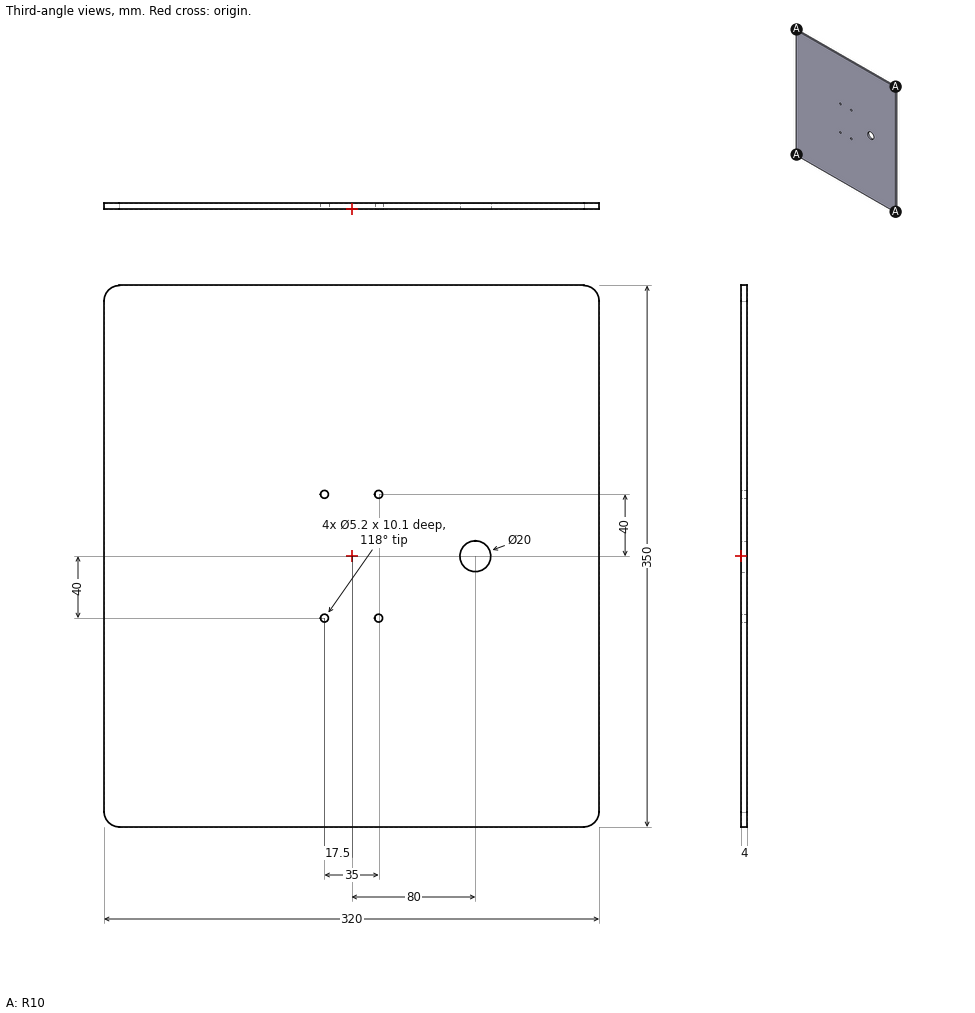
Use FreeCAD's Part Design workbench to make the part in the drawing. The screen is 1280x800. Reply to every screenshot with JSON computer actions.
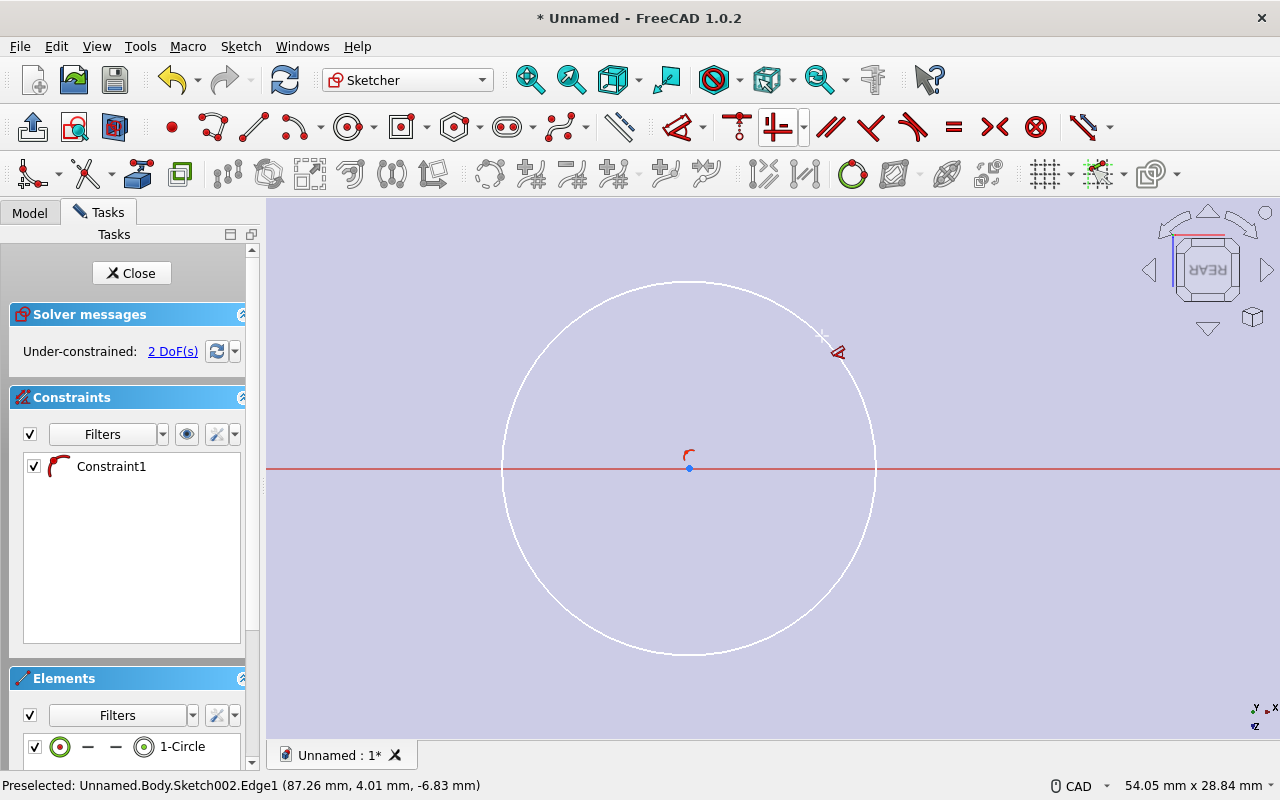
{"action": "left_click", "coordinate": [821, 336]}
{"action": "left_click", "coordinate": [844, 313]}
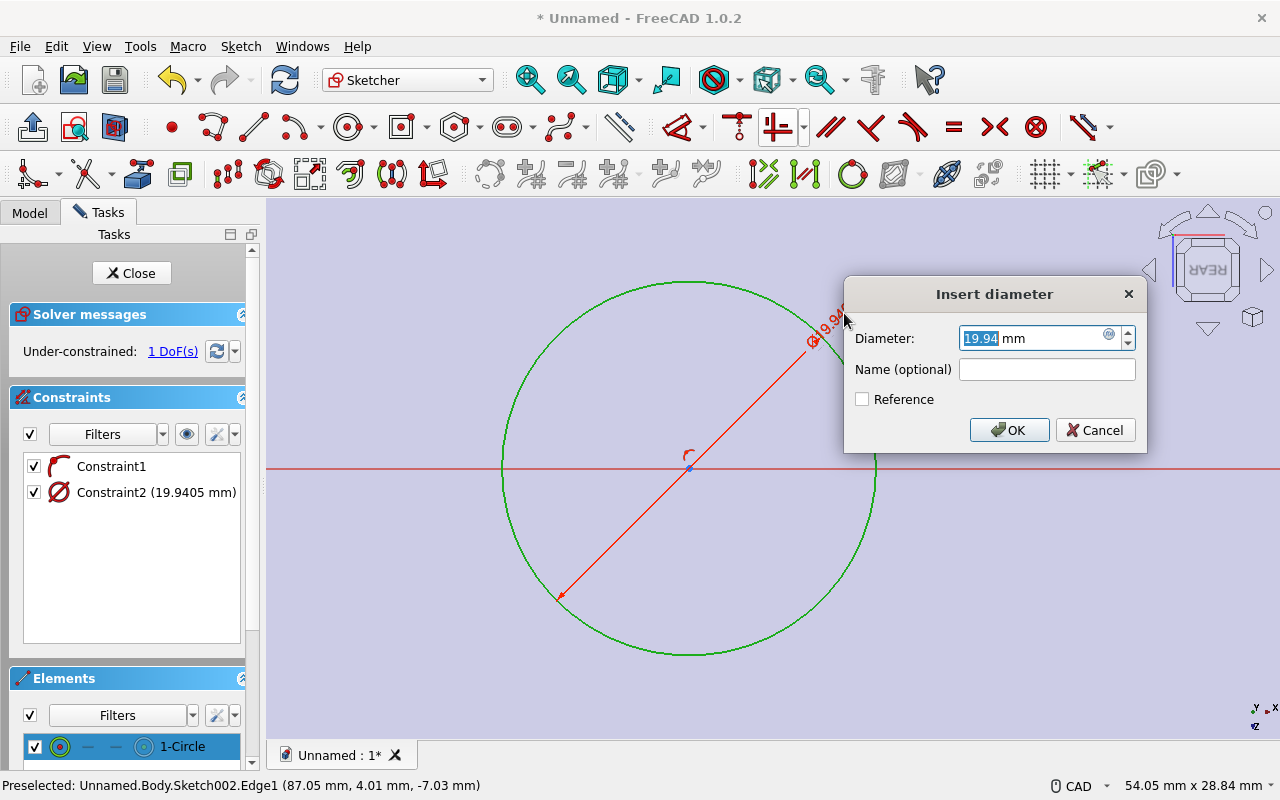
{"action": "type", "text": "20"}
{"action": "key", "text": "Return"}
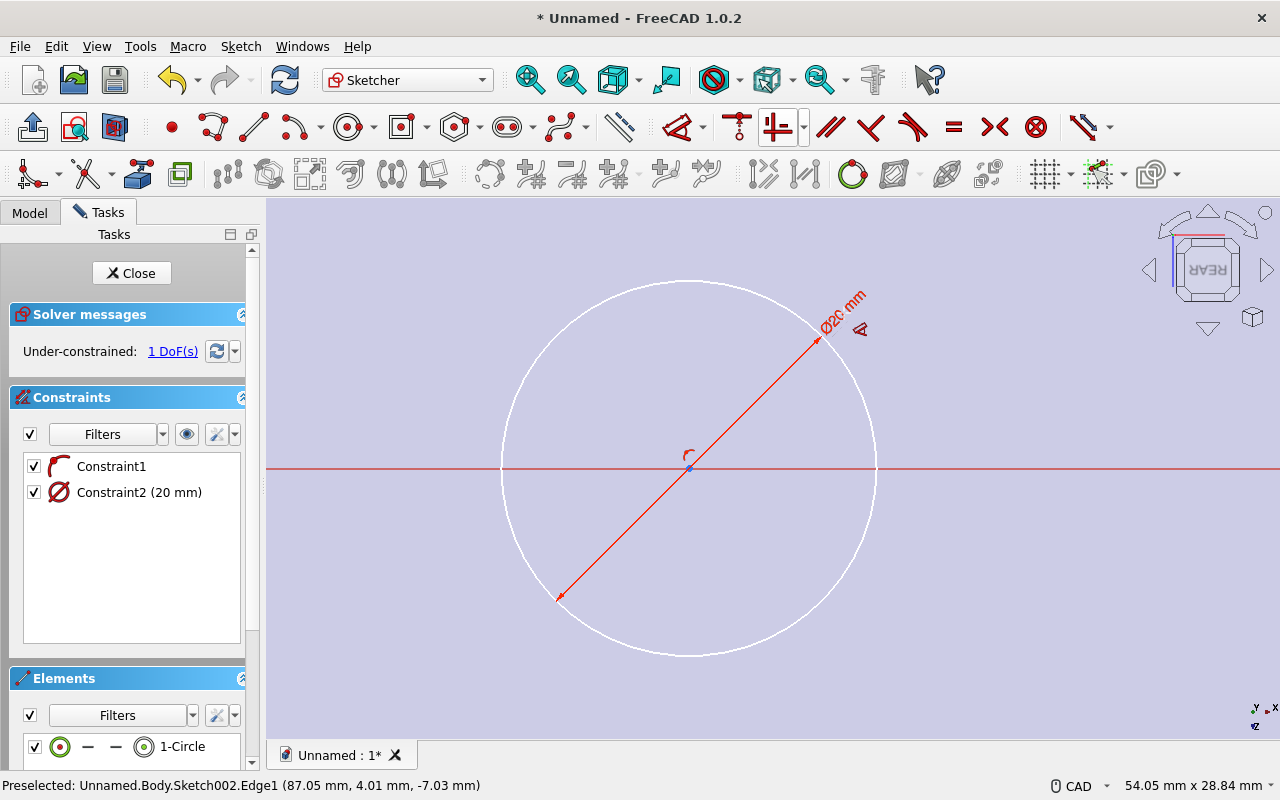
{"action": "left_click", "coordinate": [689, 468]}
{"action": "left_click", "coordinate": [401, 502]}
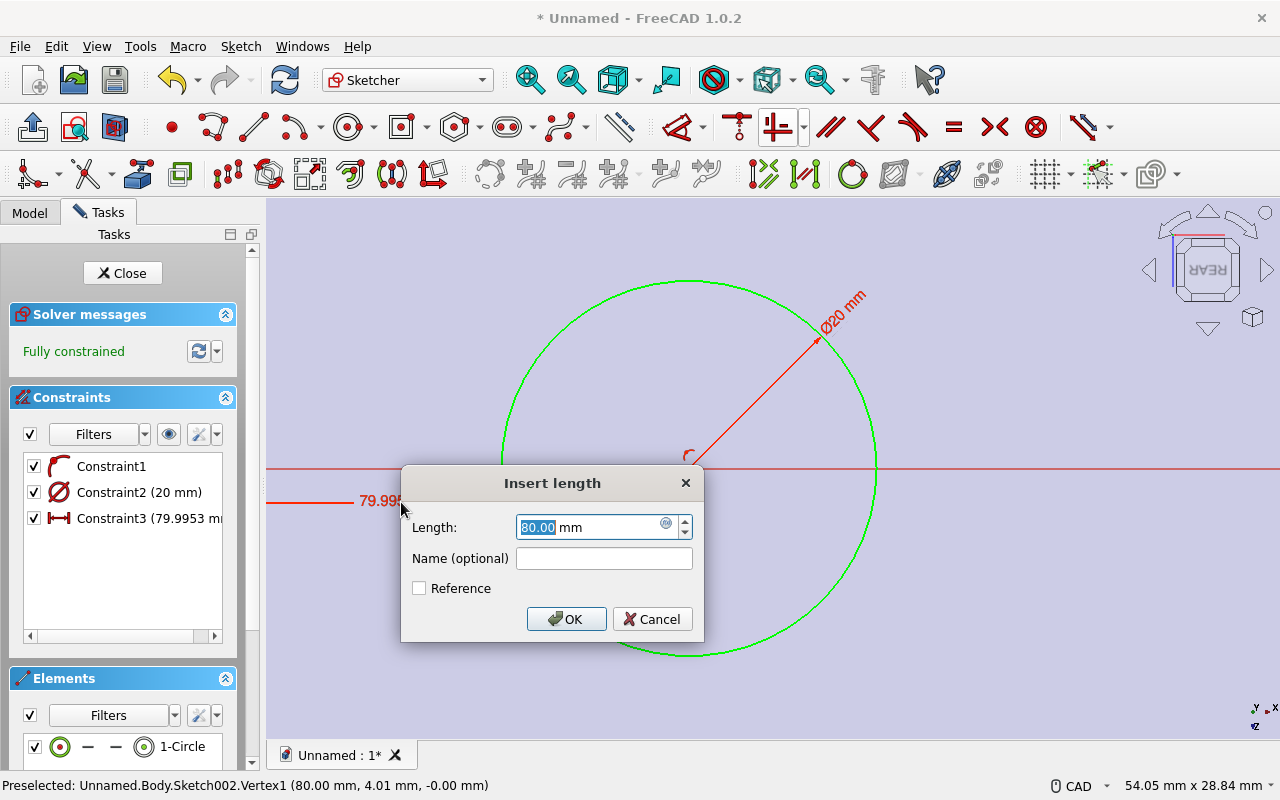
{"action": "type", "text": "80"}
{"action": "key", "text": "Return"}
{"action": "key", "text": "Escape"}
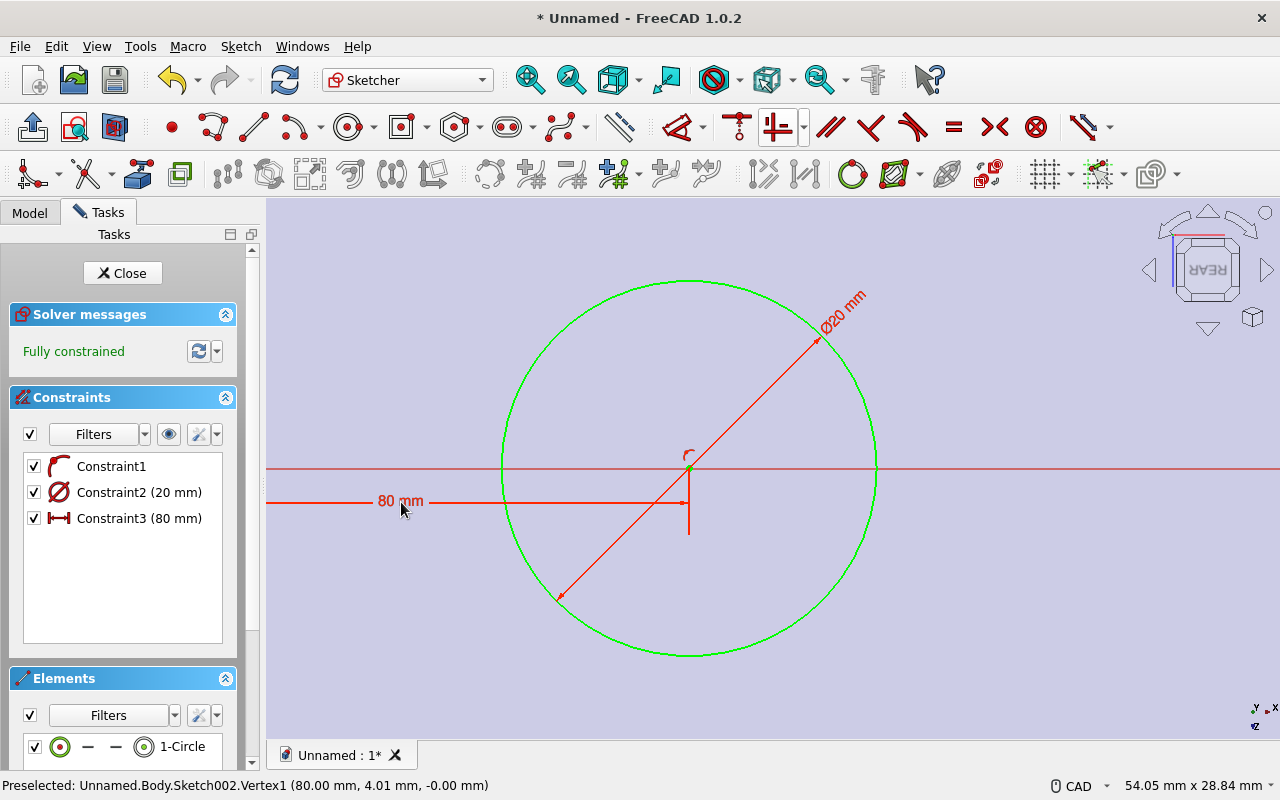
{"action": "left_click", "coordinate": [123, 273]}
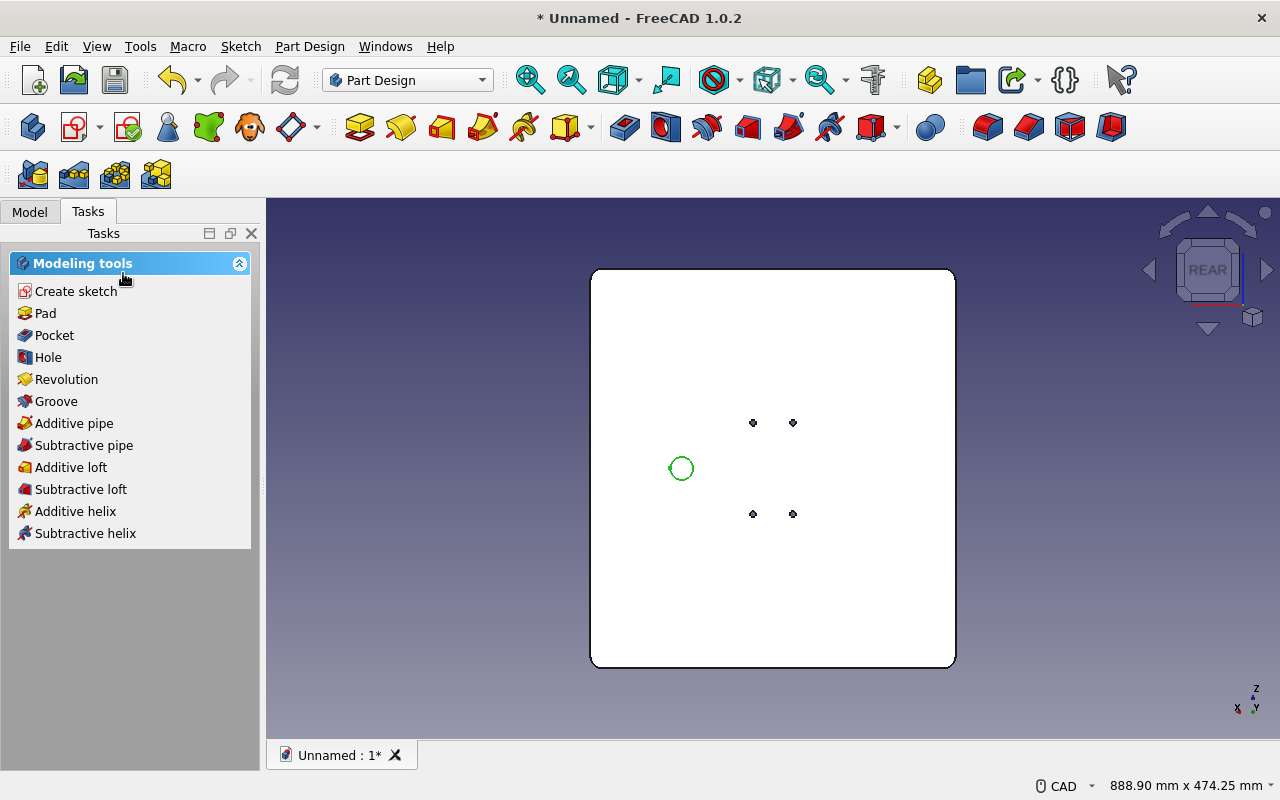
{"action": "left_click", "coordinate": [625, 128]}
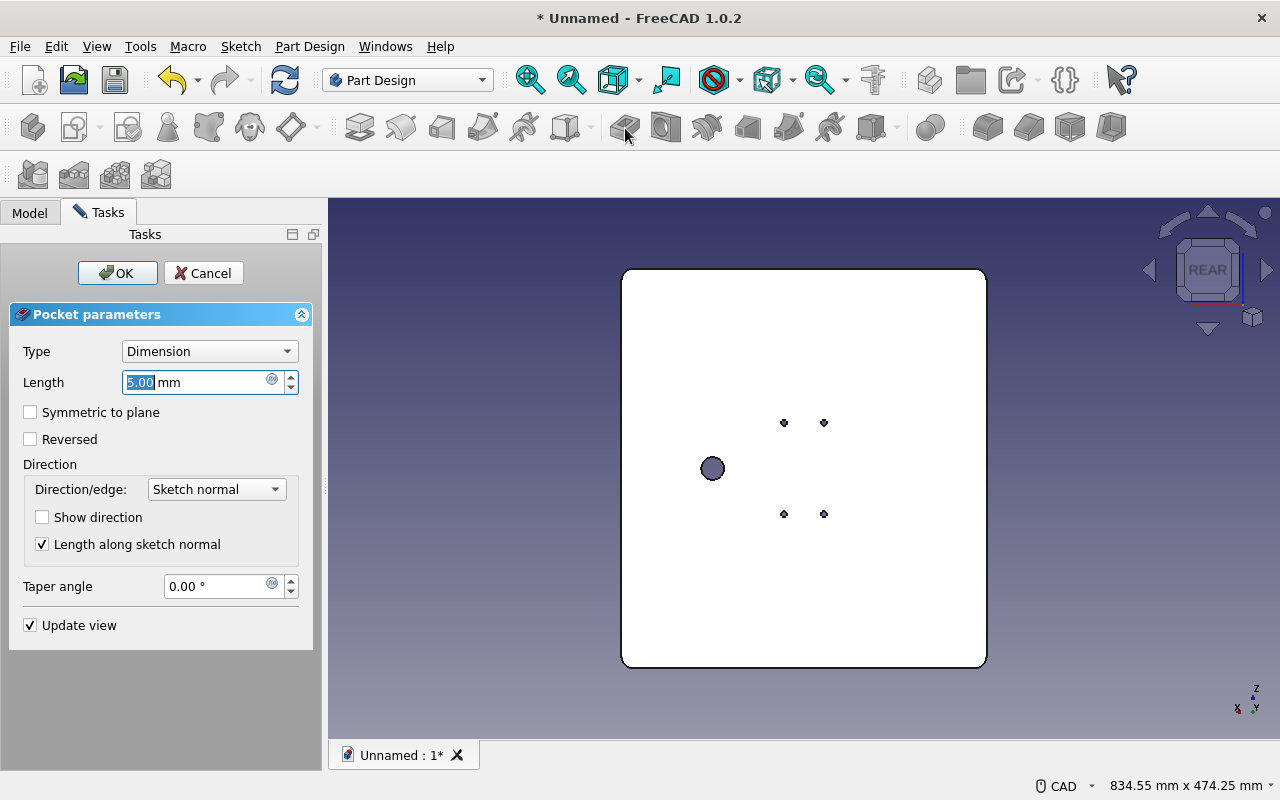
{"action": "left_click", "coordinate": [210, 352]}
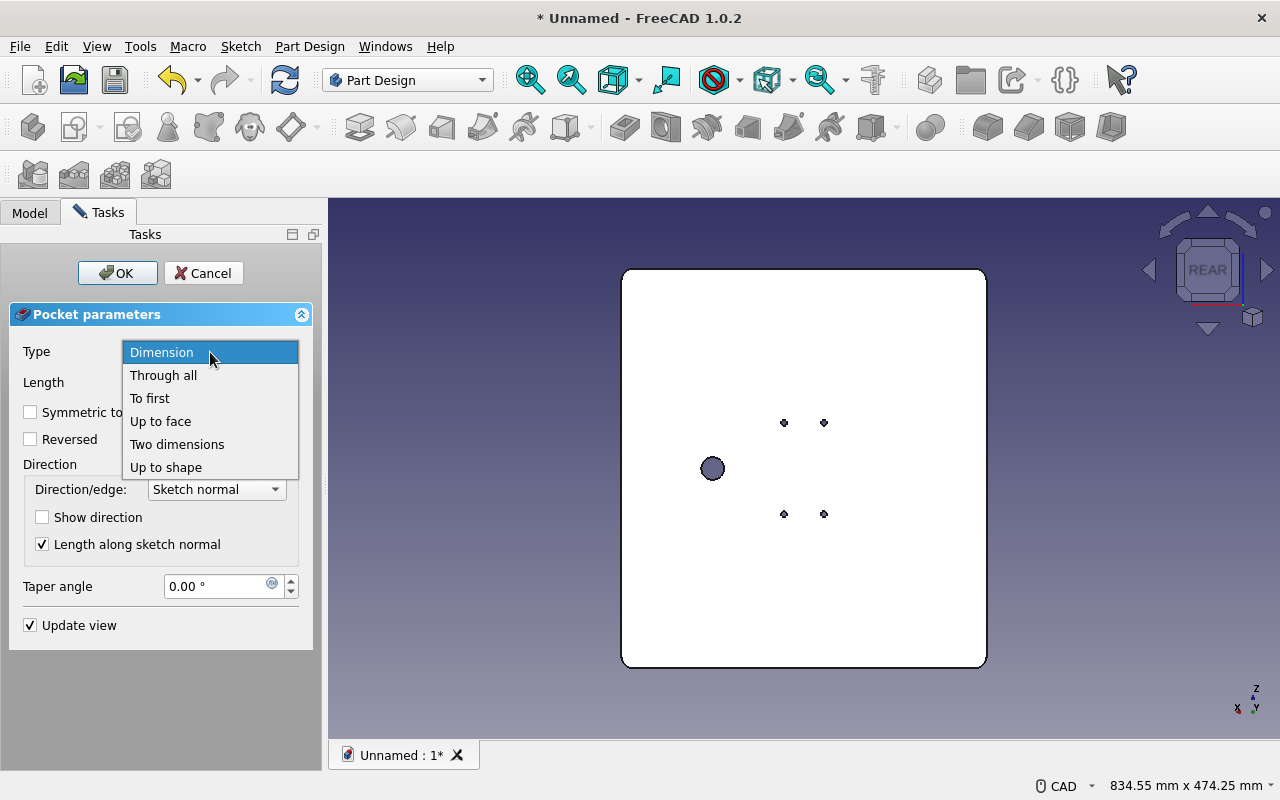
{"action": "left_click", "coordinate": [208, 376]}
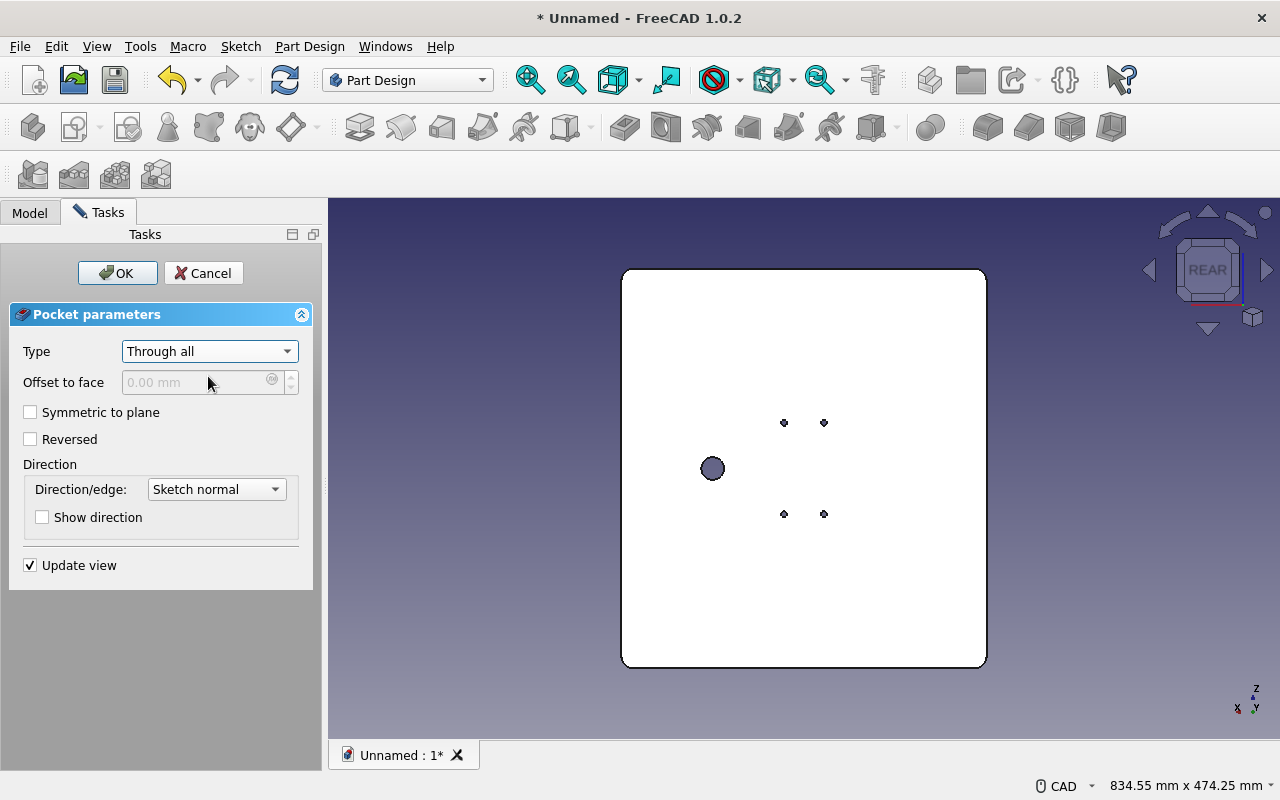
{"action": "left_click", "coordinate": [118, 273]}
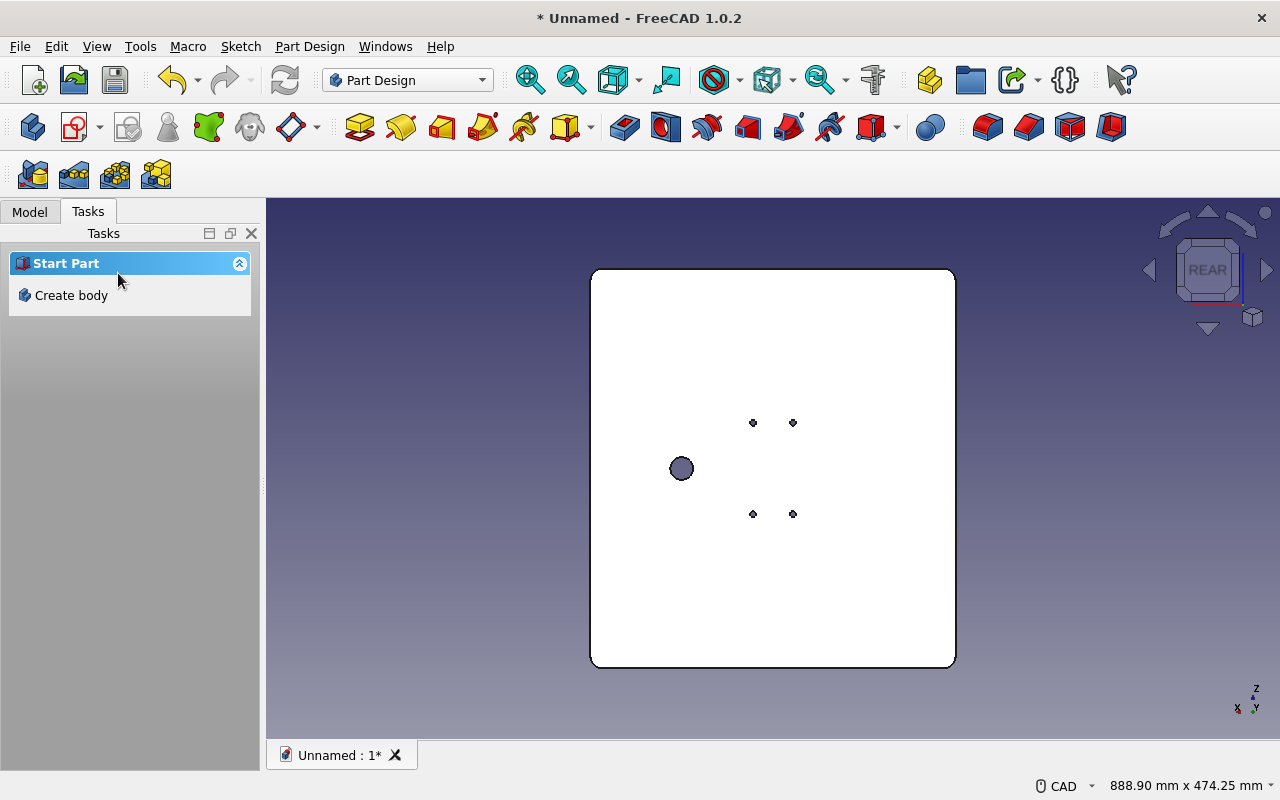
{"action": "key", "text": "0"}